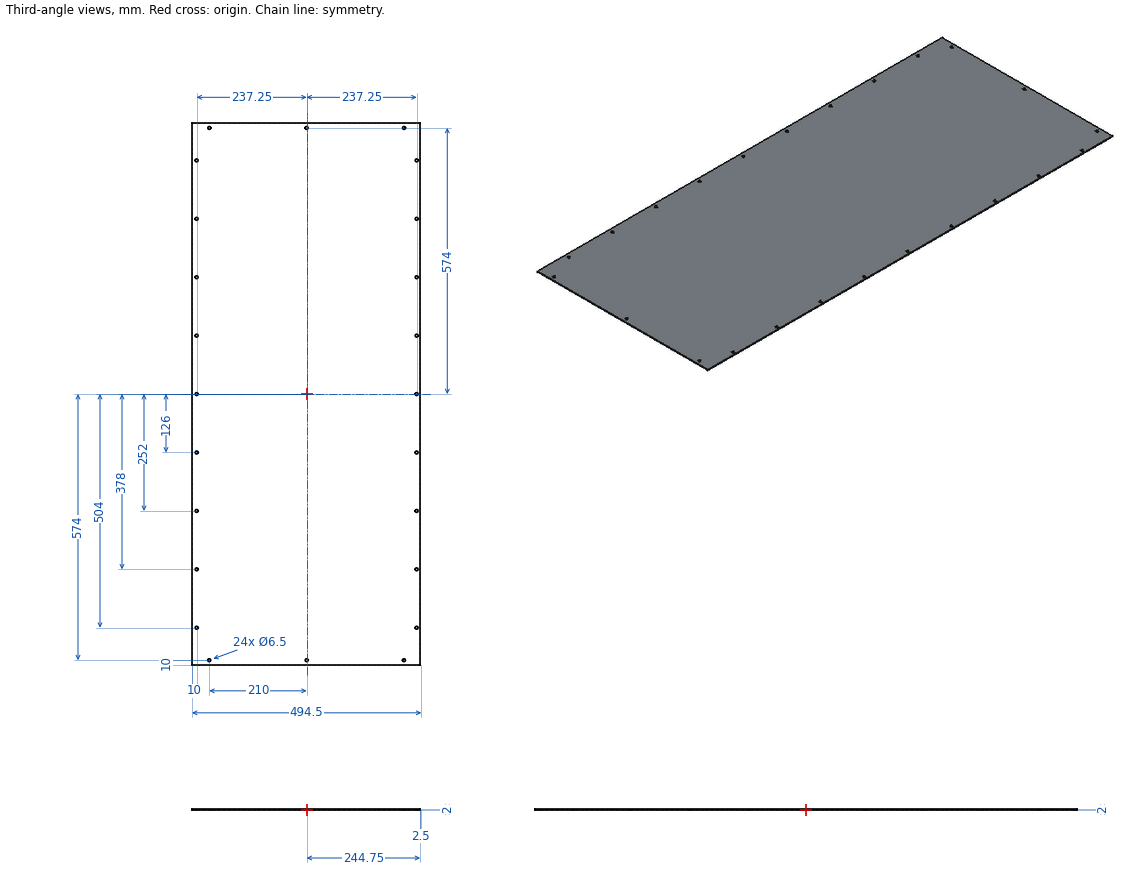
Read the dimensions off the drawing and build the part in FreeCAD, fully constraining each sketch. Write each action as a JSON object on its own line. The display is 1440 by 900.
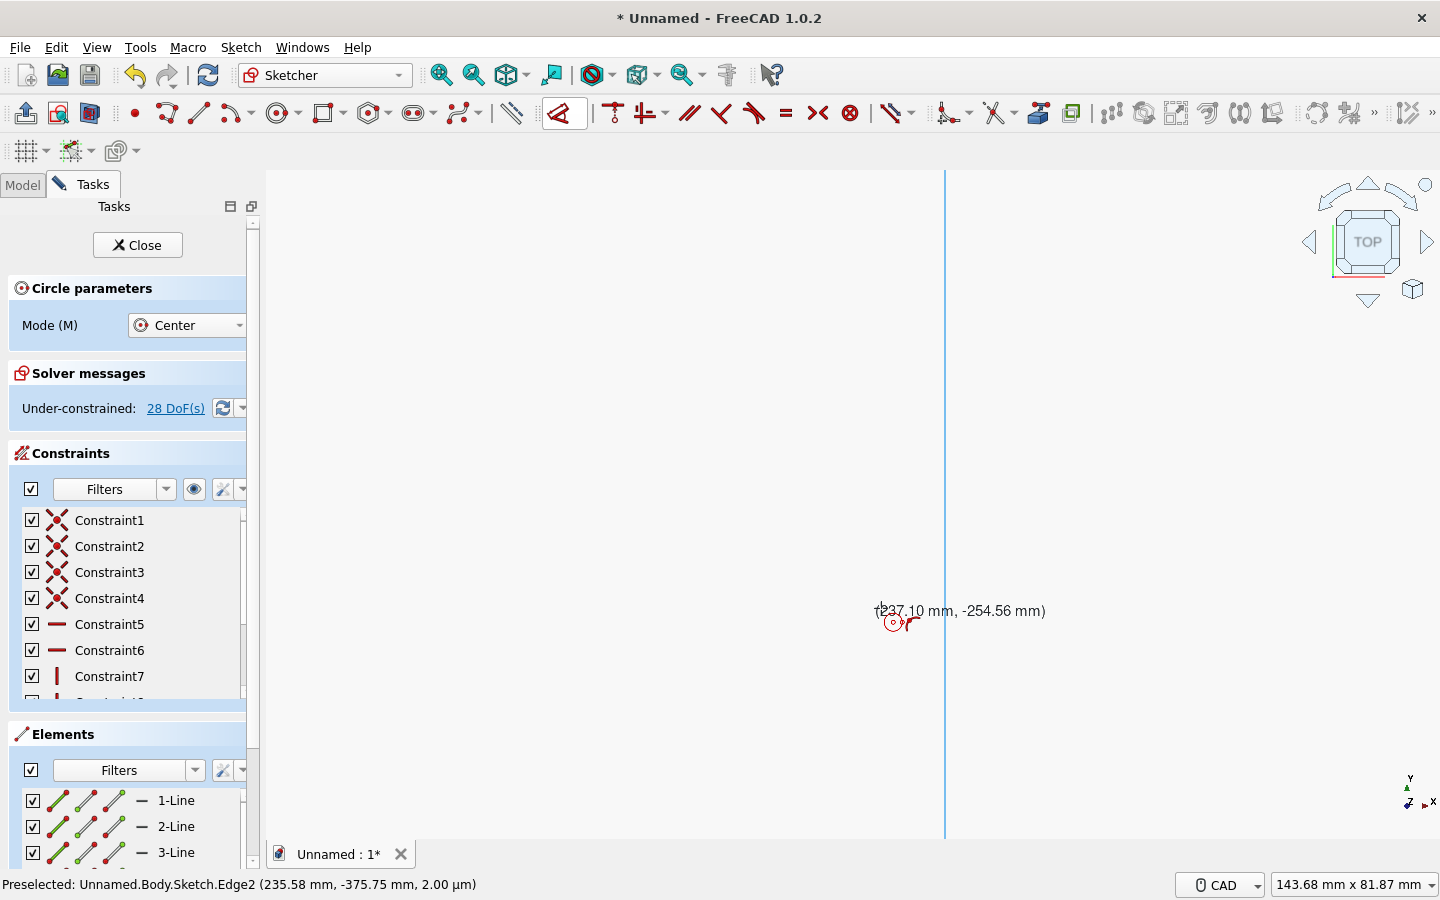
{"action": "scroll", "coordinate": [881, 608], "scroll_direction": "down", "scroll_amount": 15}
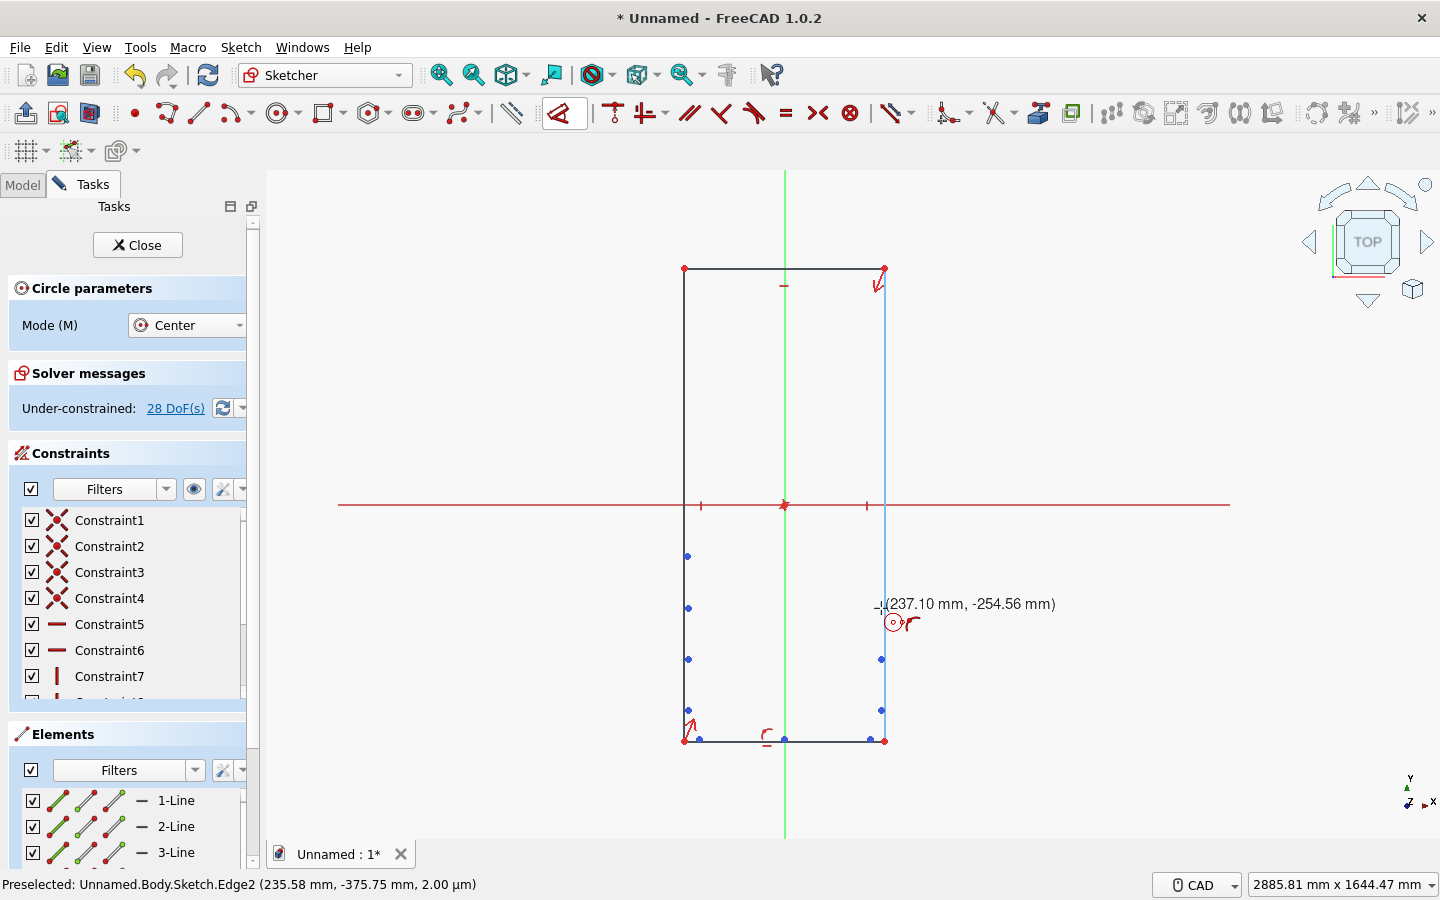
{"action": "scroll", "coordinate": [881, 608], "scroll_direction": "up", "scroll_amount": 7}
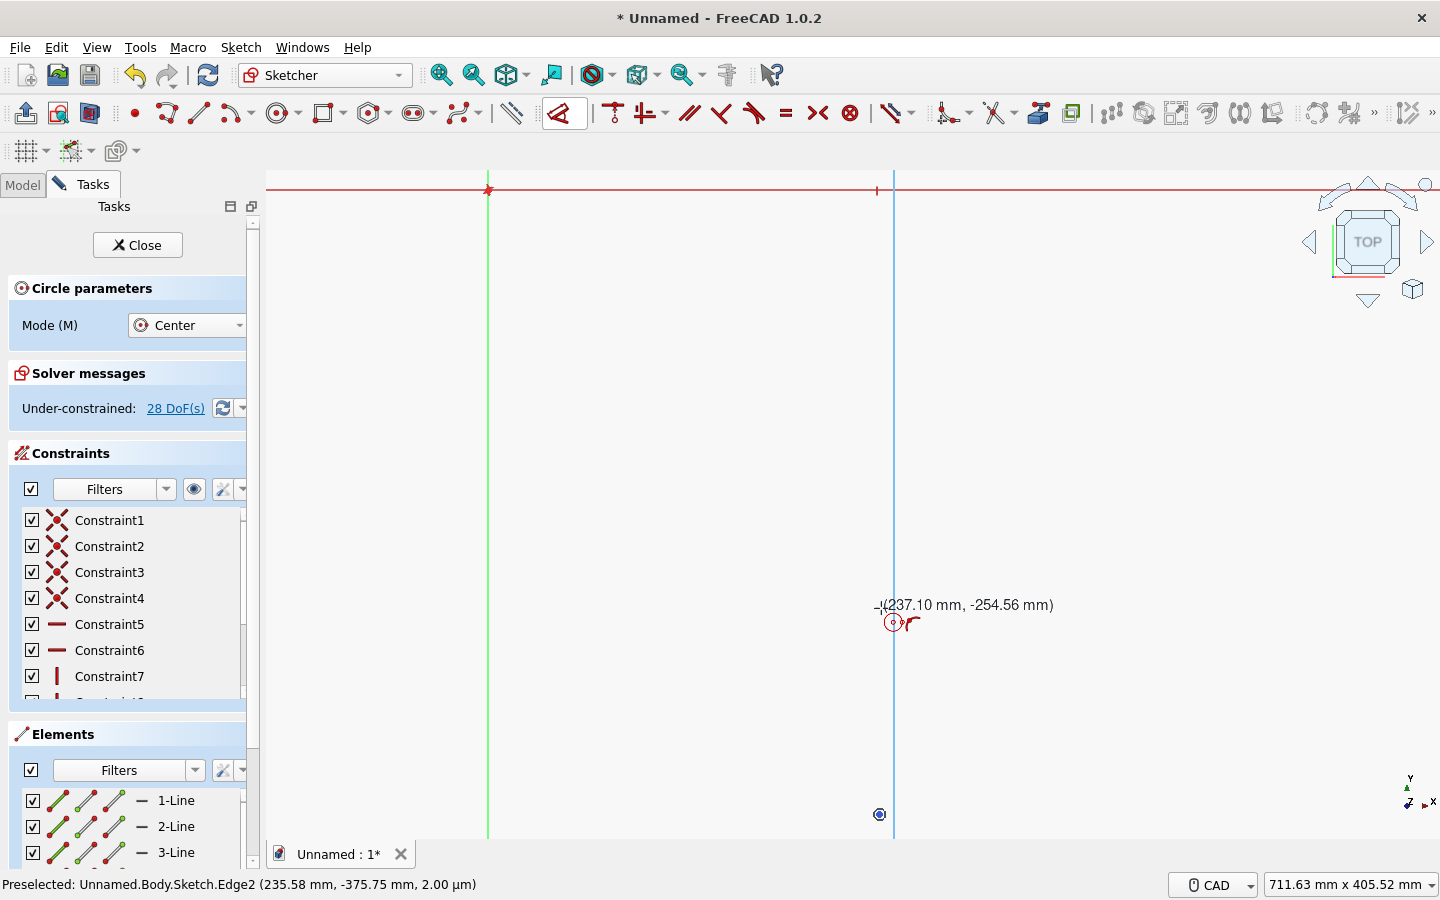
{"action": "left_click", "coordinate": [880, 606]}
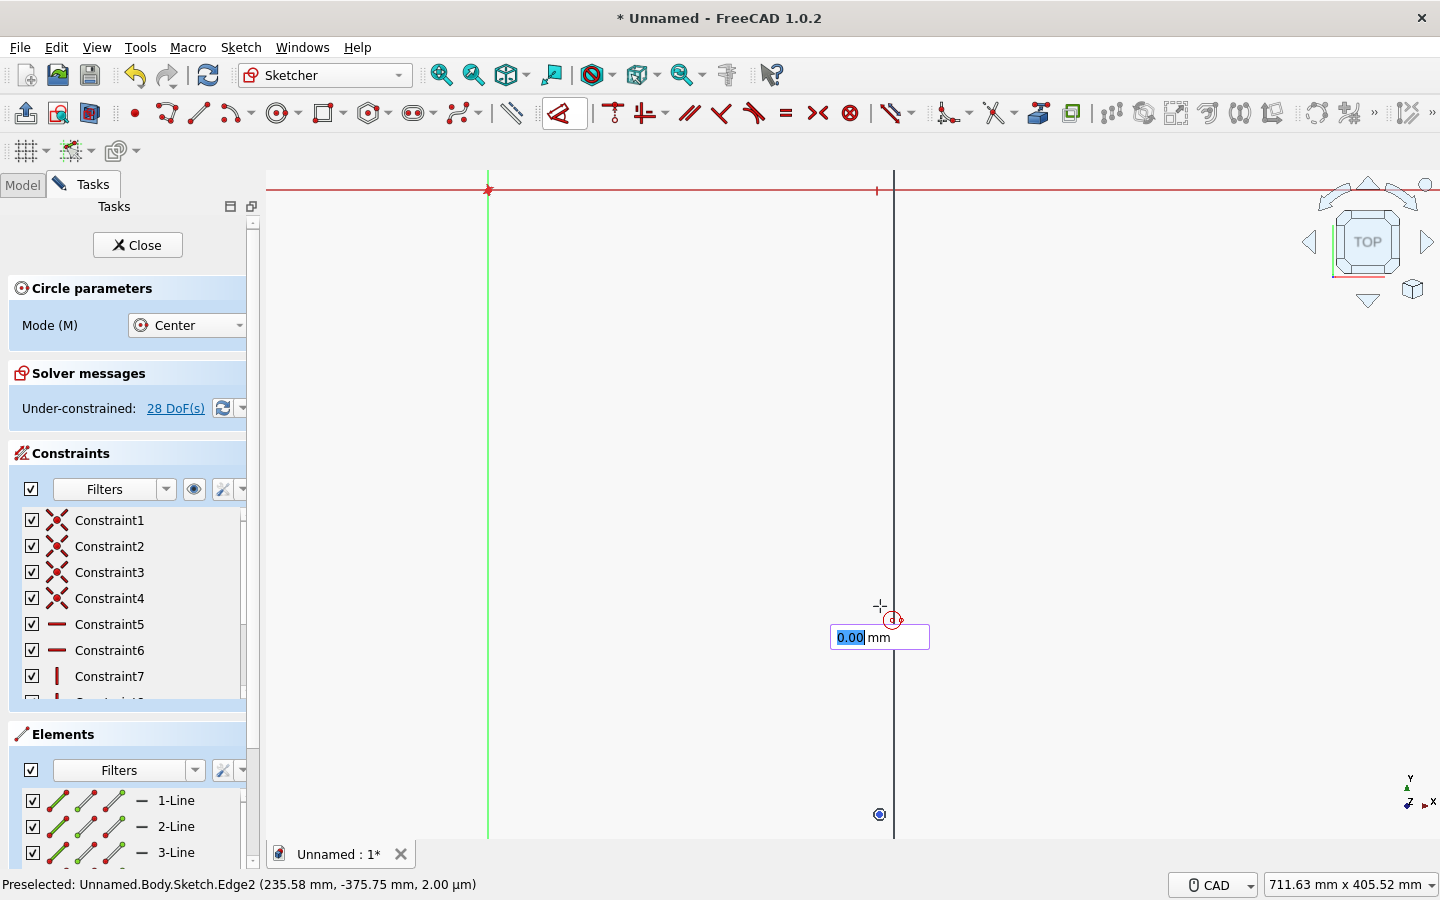
{"action": "scroll", "coordinate": [876, 602], "scroll_direction": "up", "scroll_amount": 6}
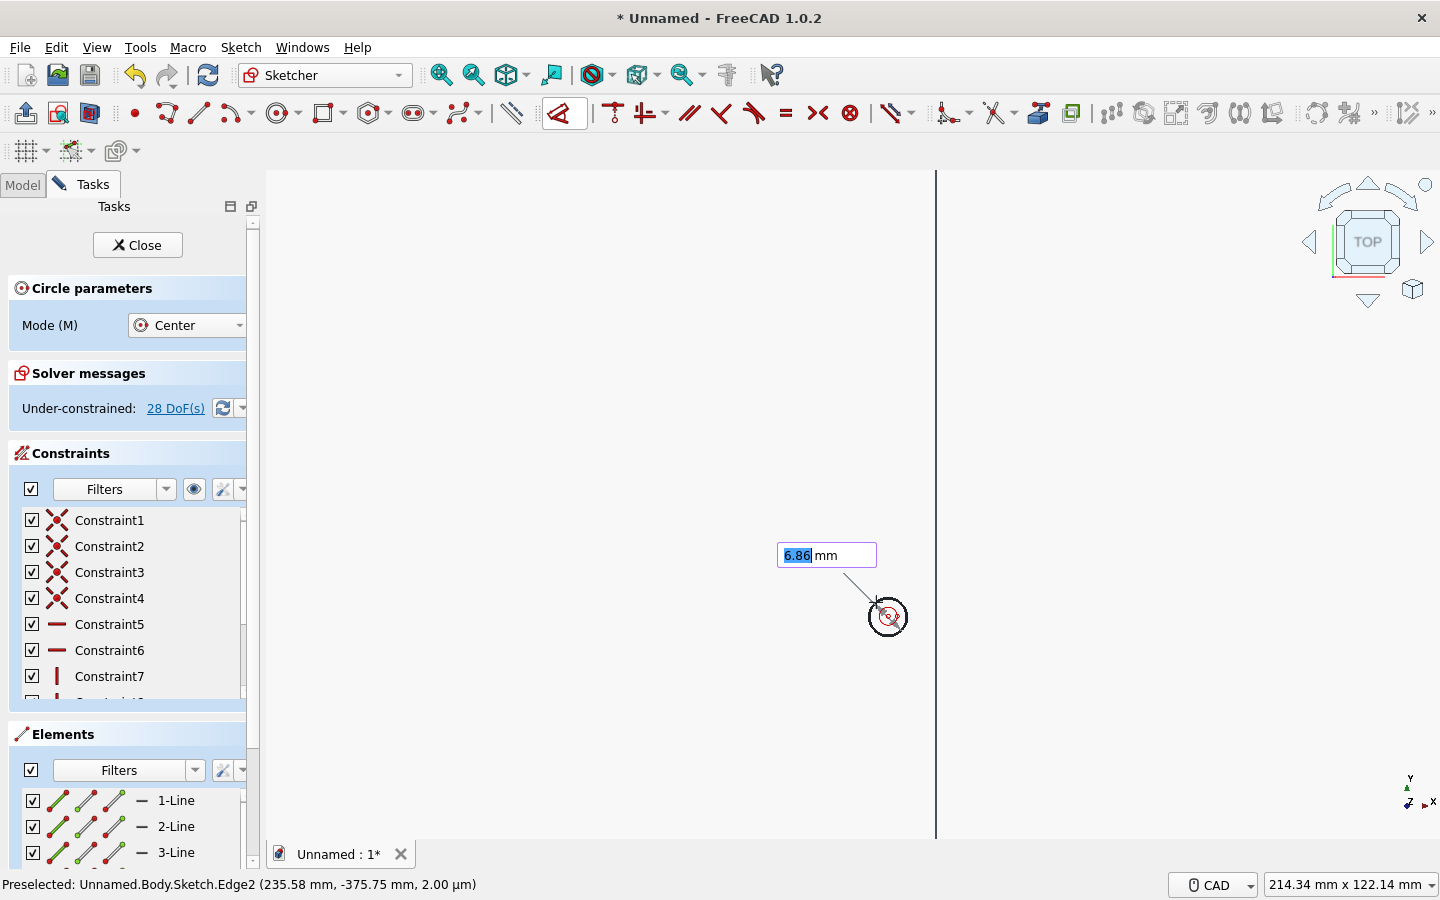
{"action": "left_click", "coordinate": [874, 601]}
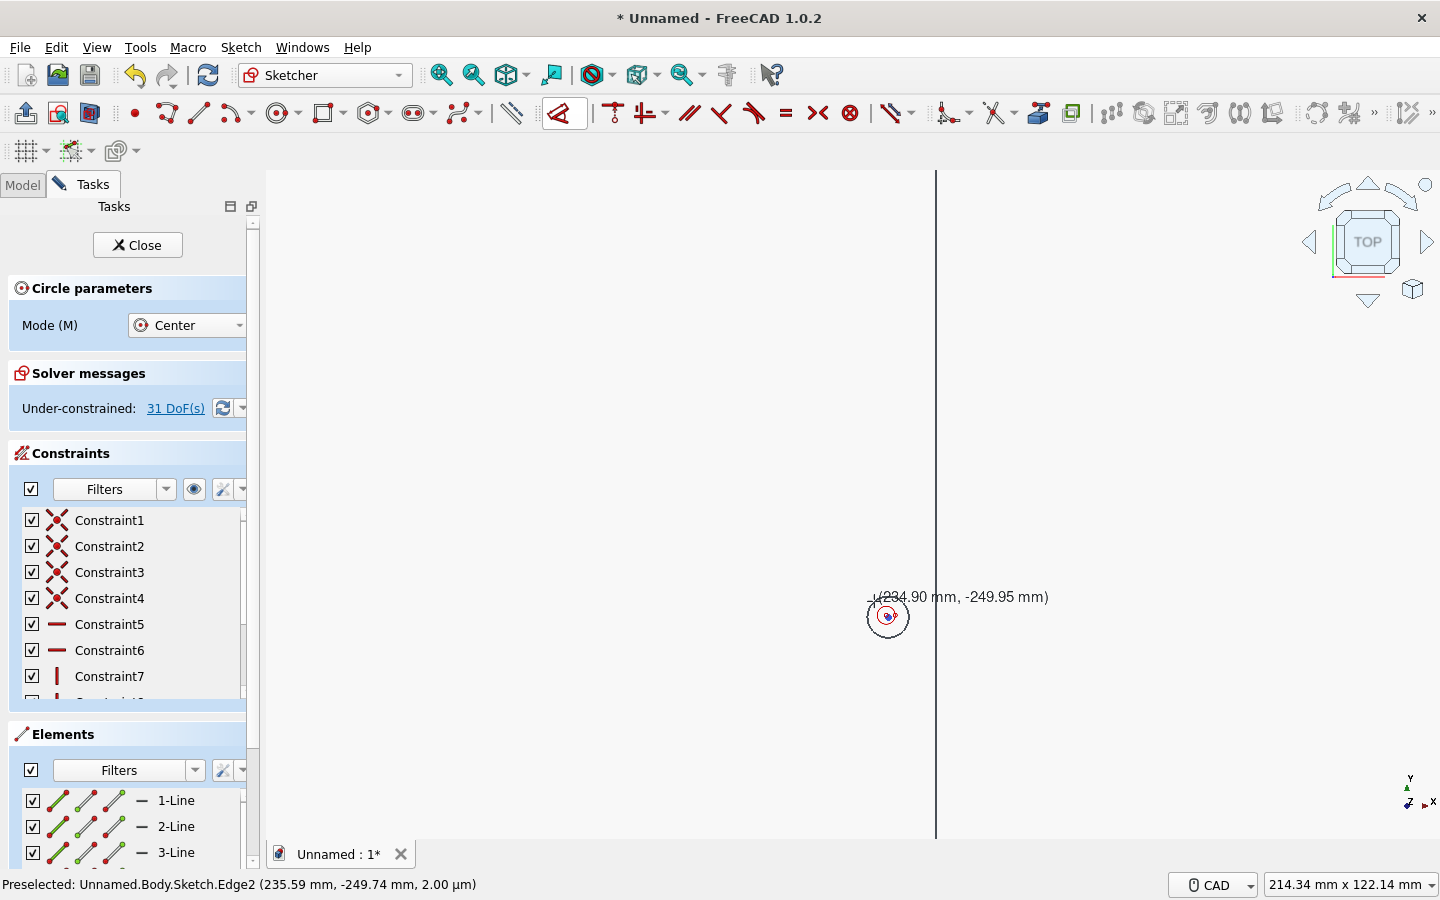
{"action": "scroll", "coordinate": [881, 607], "scroll_direction": "down", "scroll_amount": 13}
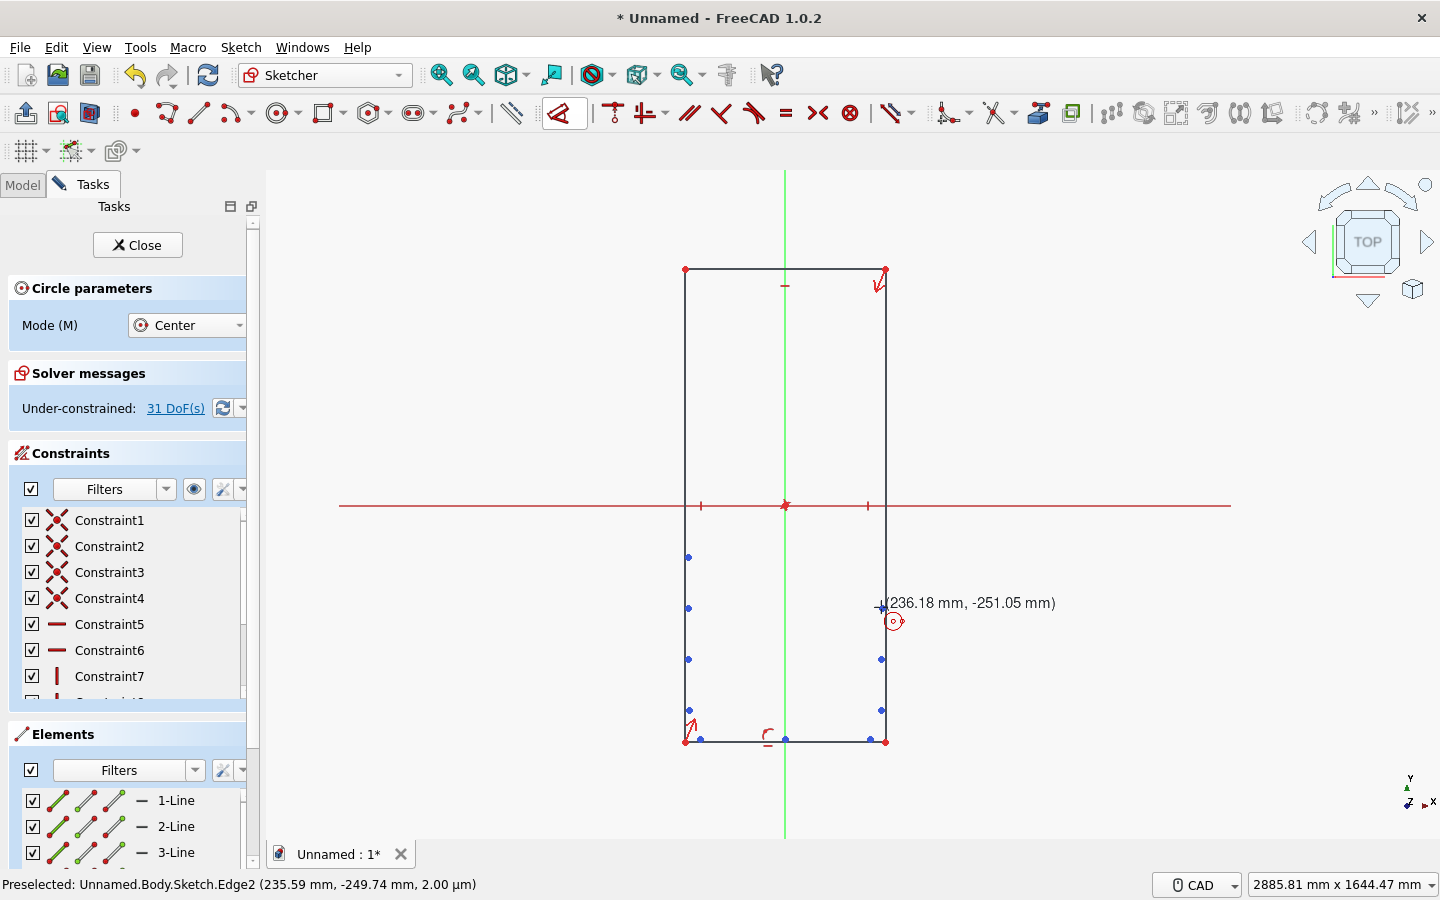
{"action": "scroll", "coordinate": [882, 557], "scroll_direction": "up", "scroll_amount": 15}